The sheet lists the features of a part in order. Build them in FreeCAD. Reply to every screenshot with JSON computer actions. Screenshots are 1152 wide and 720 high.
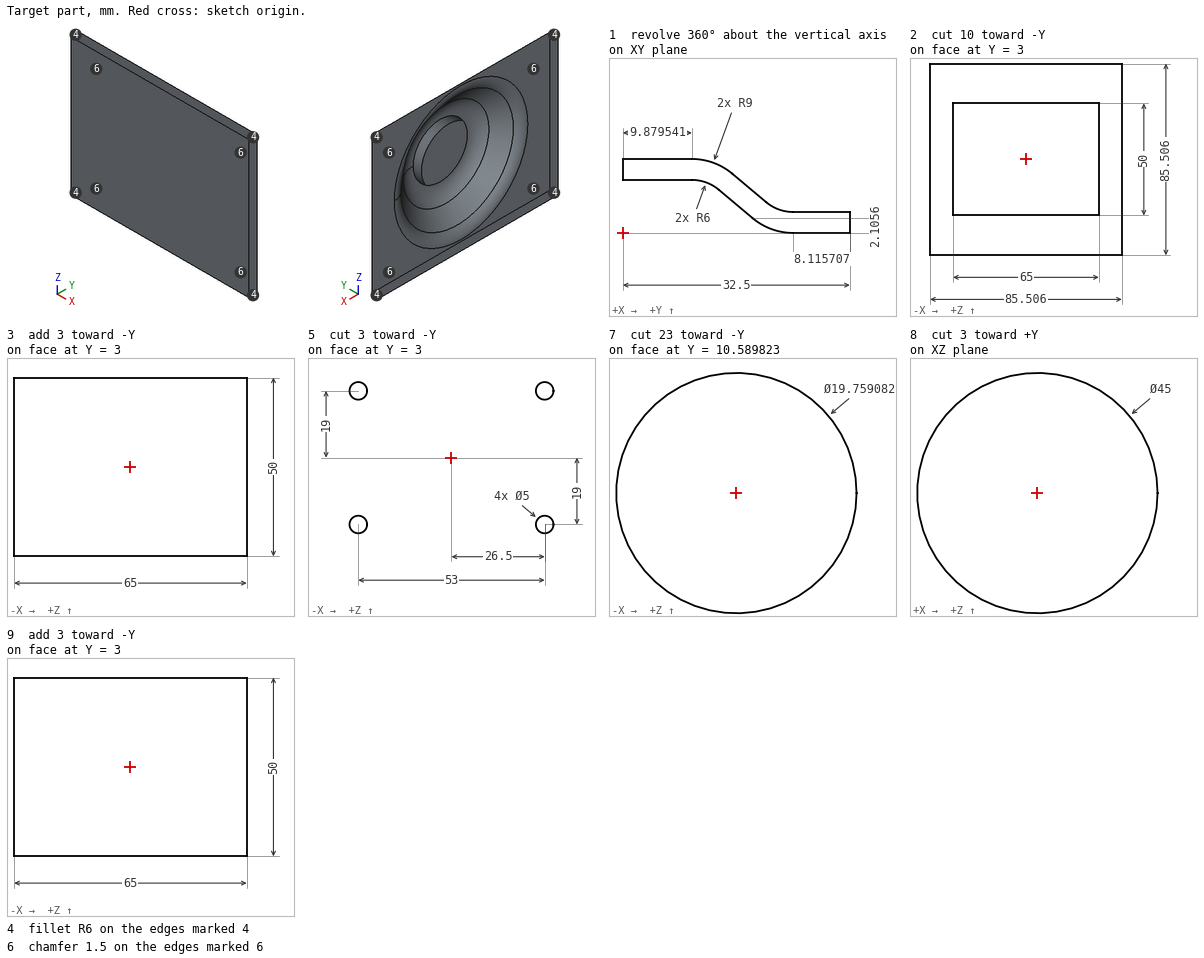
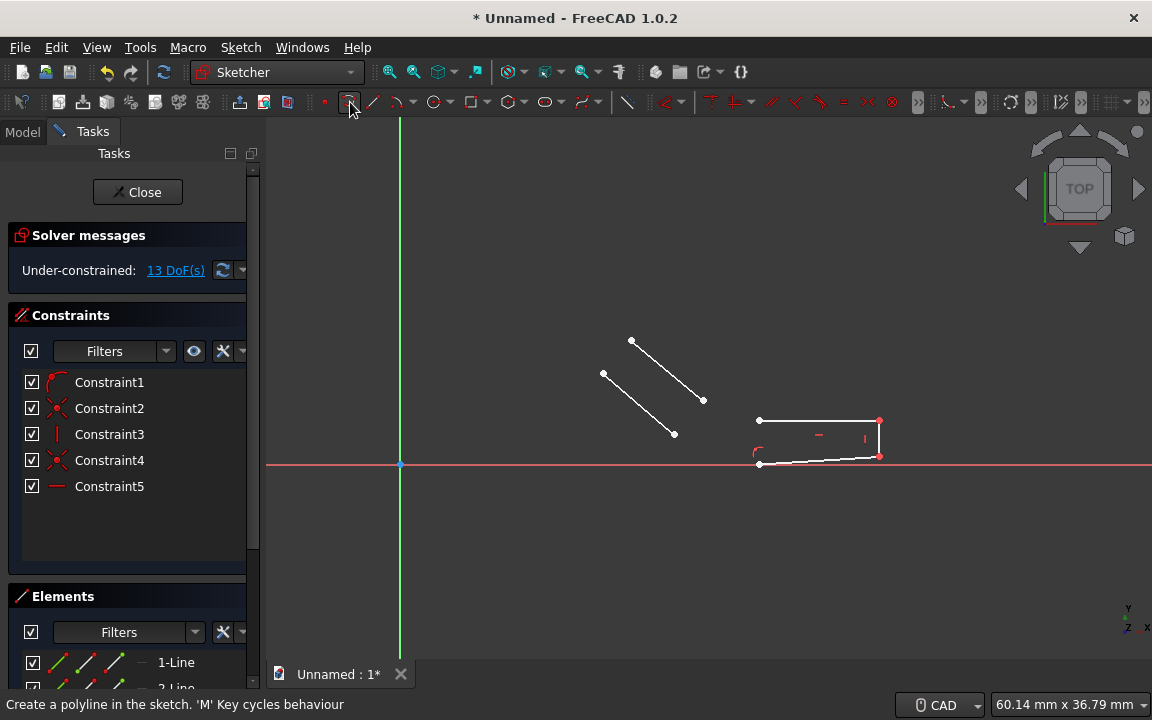
{"action": "left_click", "coordinate": [546, 309]}
{"action": "left_click", "coordinate": [400, 309]}
{"action": "left_click", "coordinate": [409, 353]}
{"action": "left_click", "coordinate": [546, 353]}
{"action": "right_click", "coordinate": [546, 353]}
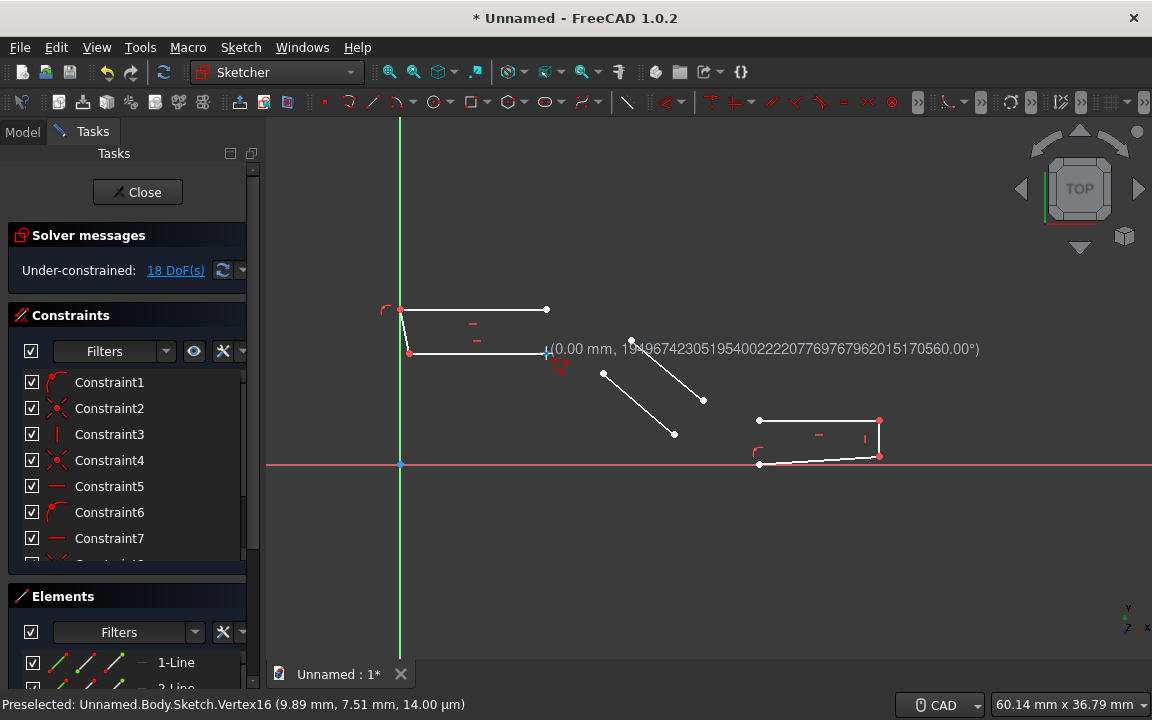
{"action": "left_click", "coordinate": [416, 102]}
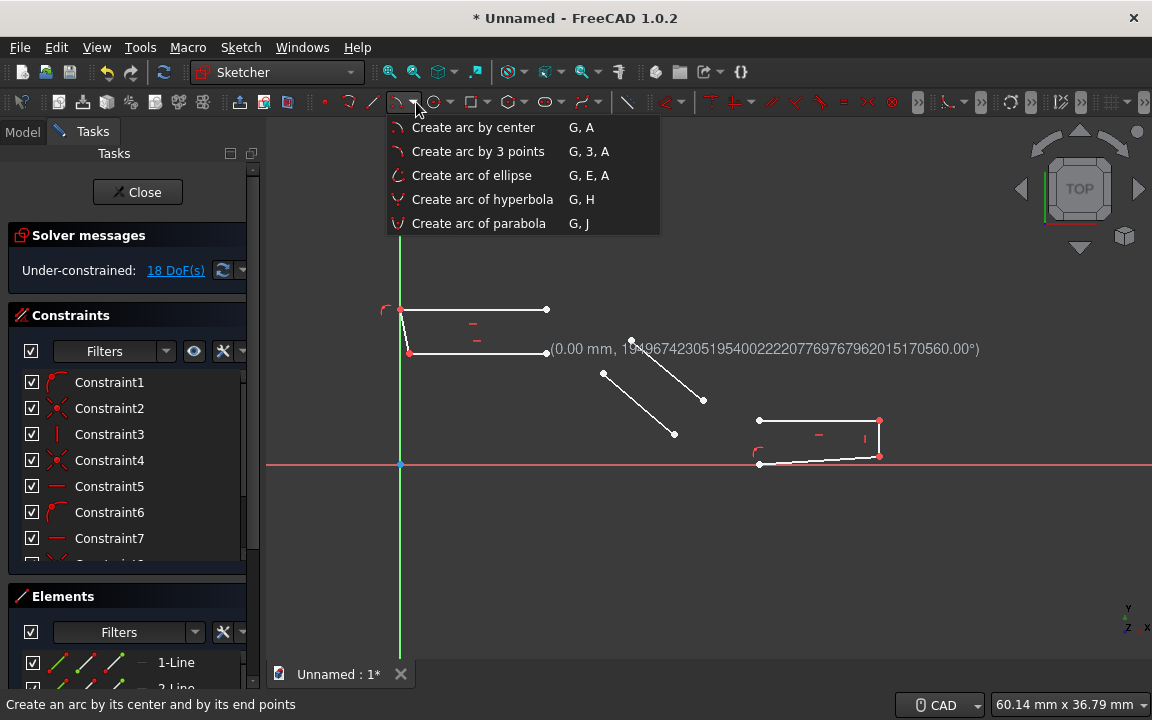
{"action": "left_click", "coordinate": [524, 151]}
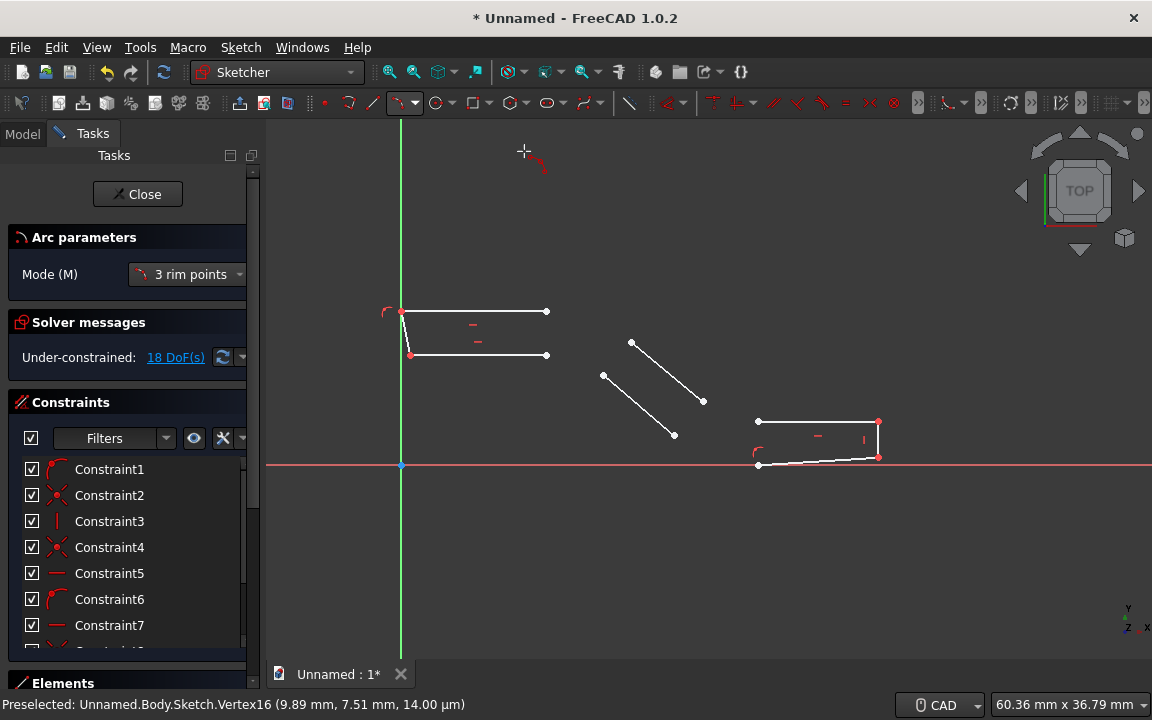
{"action": "left_click", "coordinate": [674, 436]}
{"action": "left_click", "coordinate": [759, 465]}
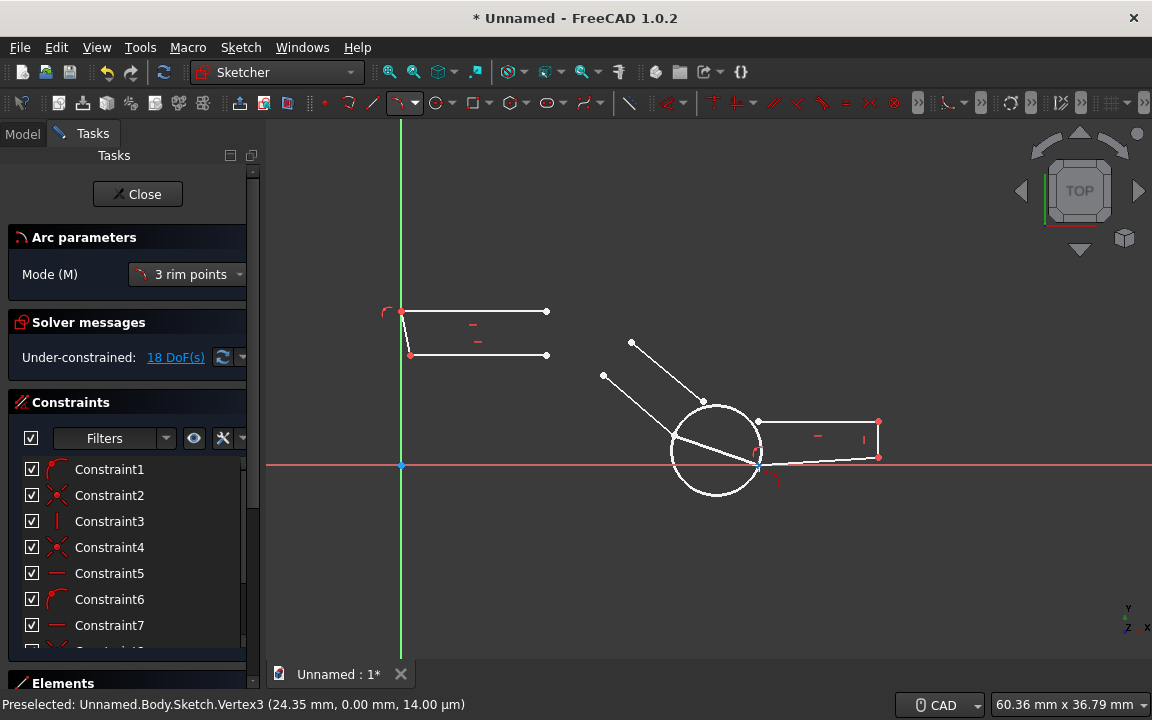
{"action": "scroll", "coordinate": [714, 457], "scroll_direction": "up", "scroll_amount": 4}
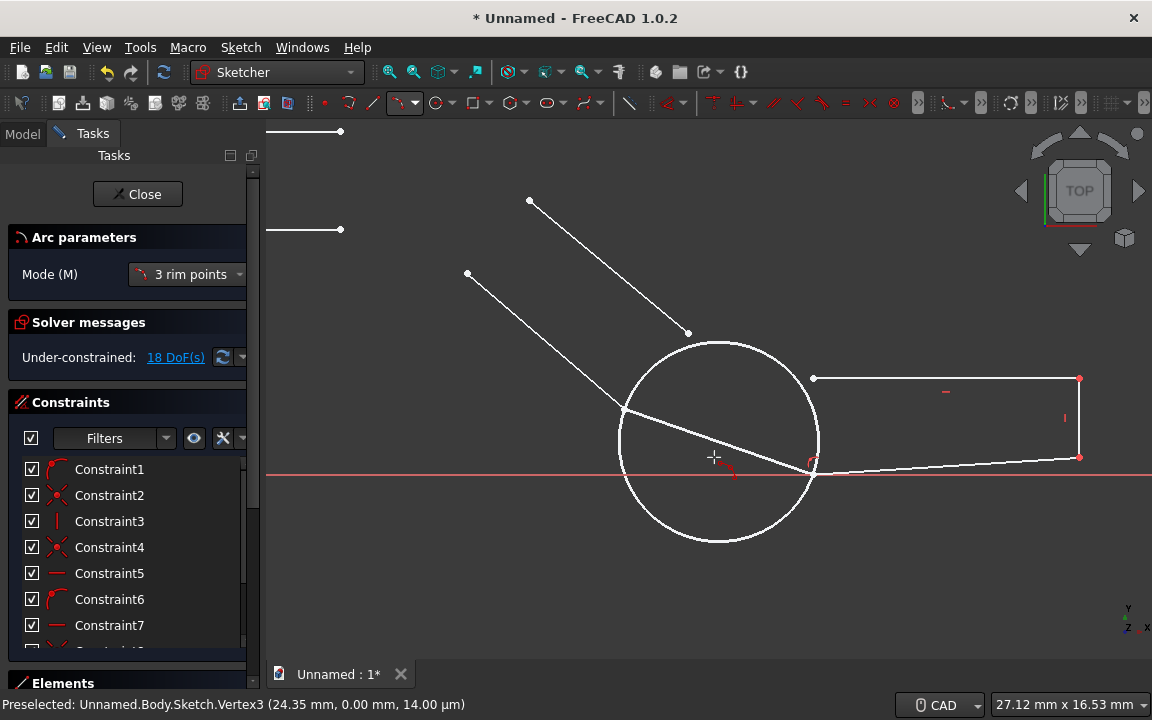
{"action": "left_click", "coordinate": [714, 457]}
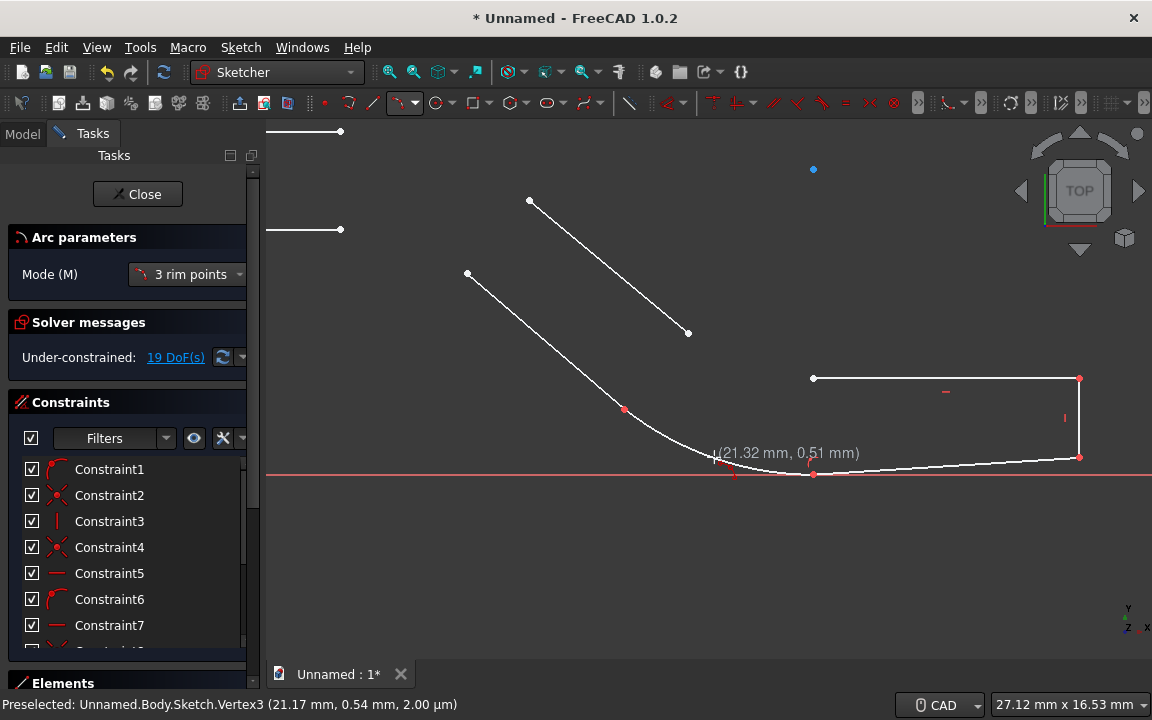
{"action": "left_click", "coordinate": [813, 378]}
{"action": "left_click", "coordinate": [689, 334]}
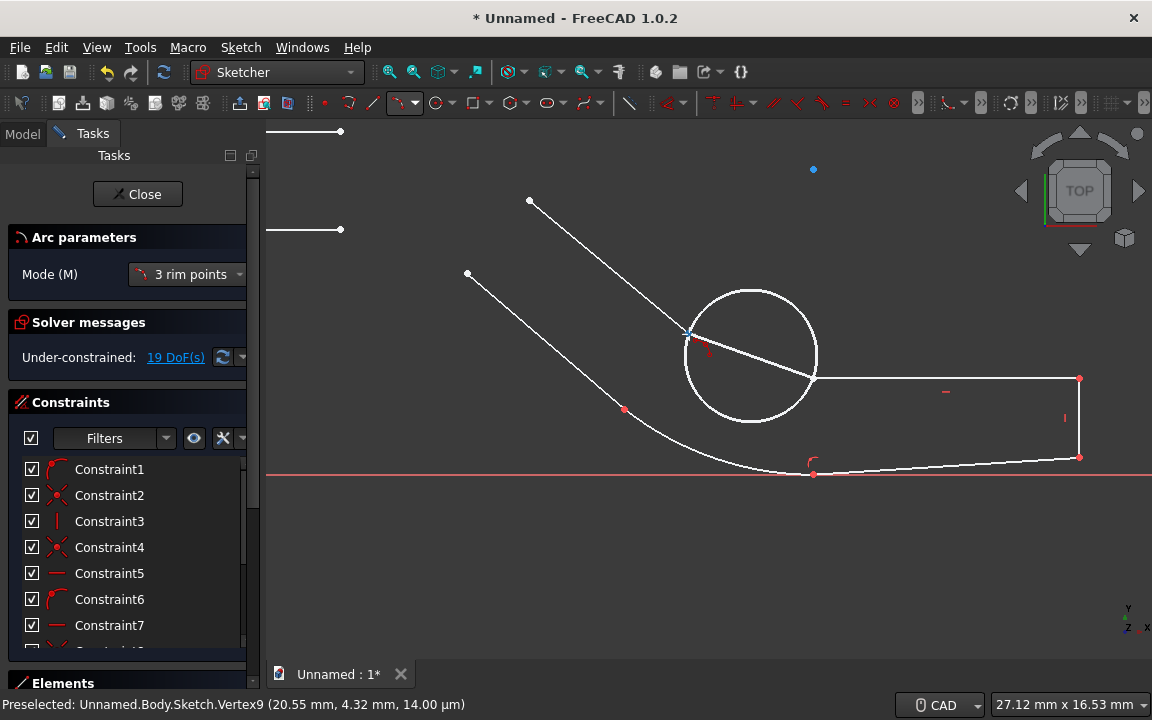
{"action": "scroll", "coordinate": [747, 365], "scroll_direction": "up", "scroll_amount": 2}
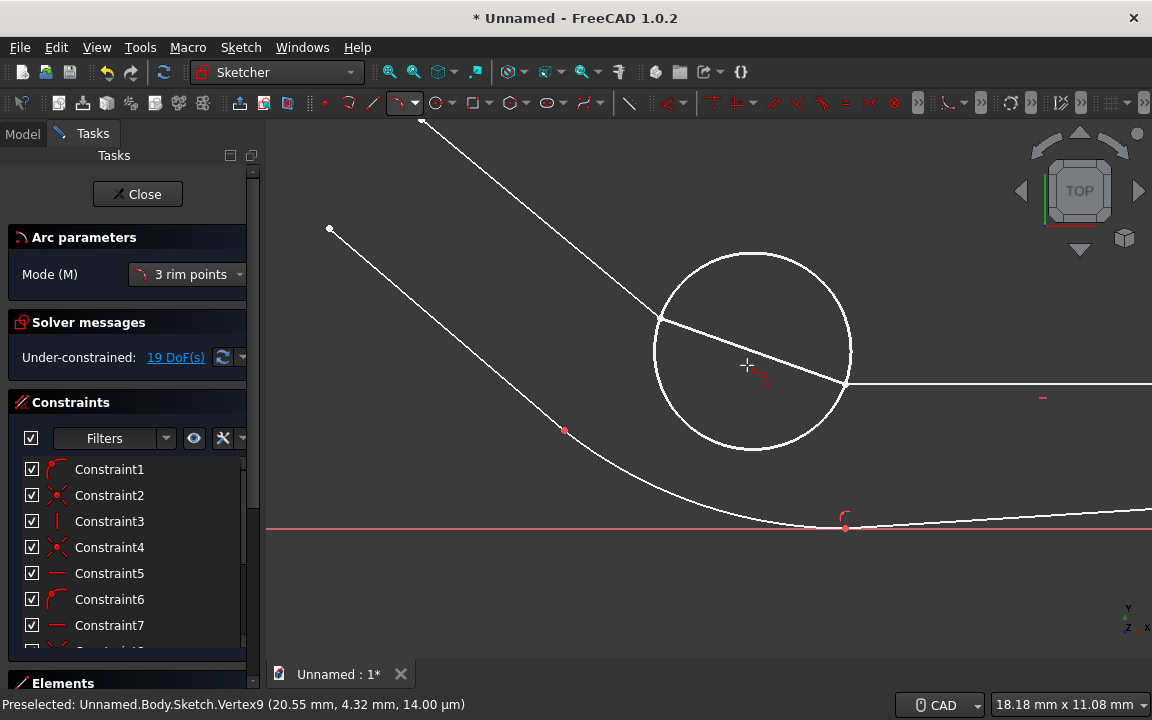
{"action": "left_click", "coordinate": [747, 365]}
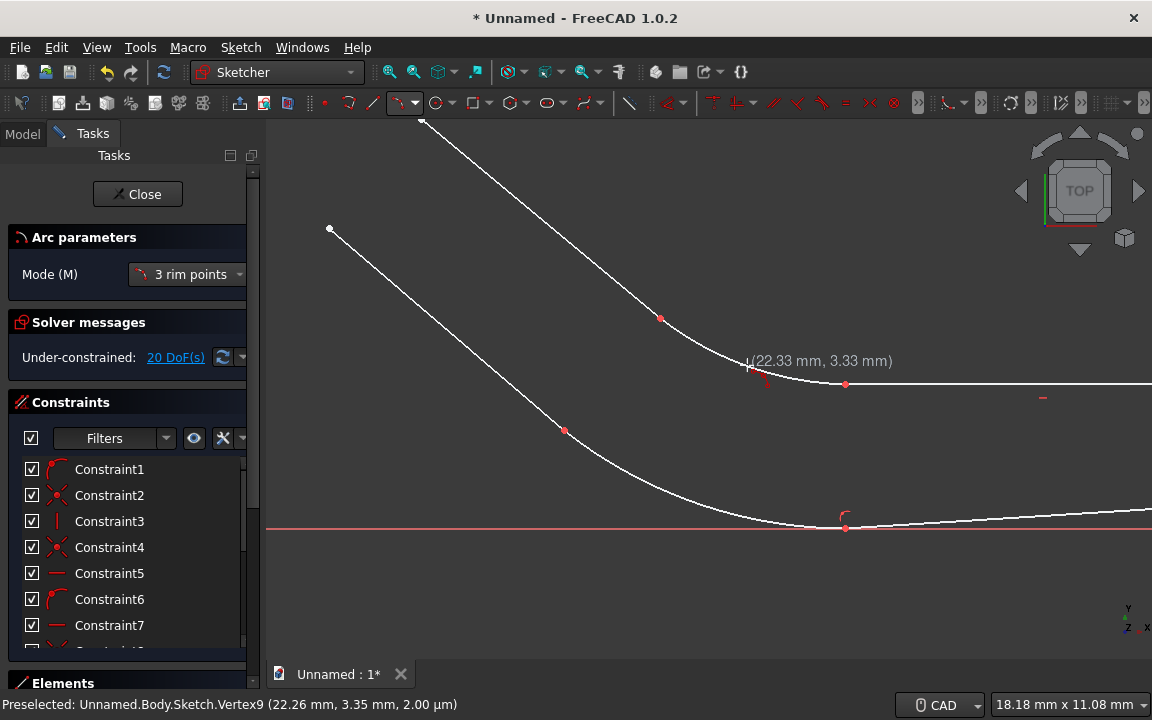
{"action": "scroll", "coordinate": [722, 440], "scroll_direction": "down", "scroll_amount": 6}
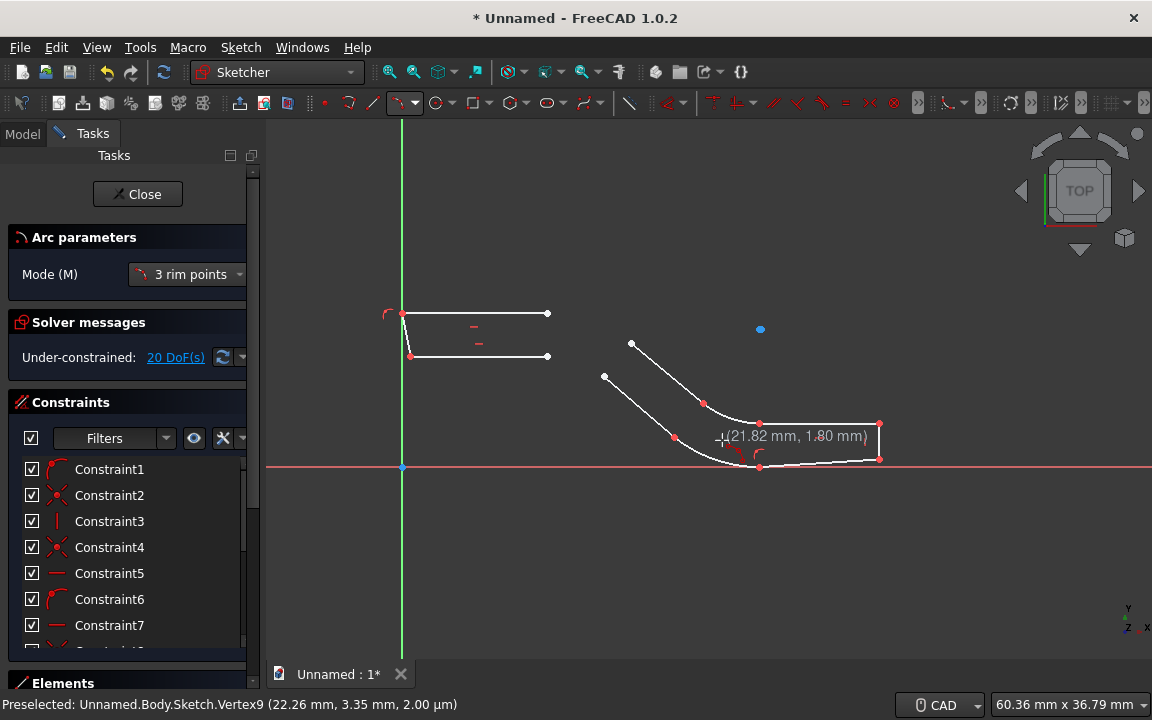
{"action": "left_click", "coordinate": [632, 344]}
{"action": "left_click", "coordinate": [547, 313]}